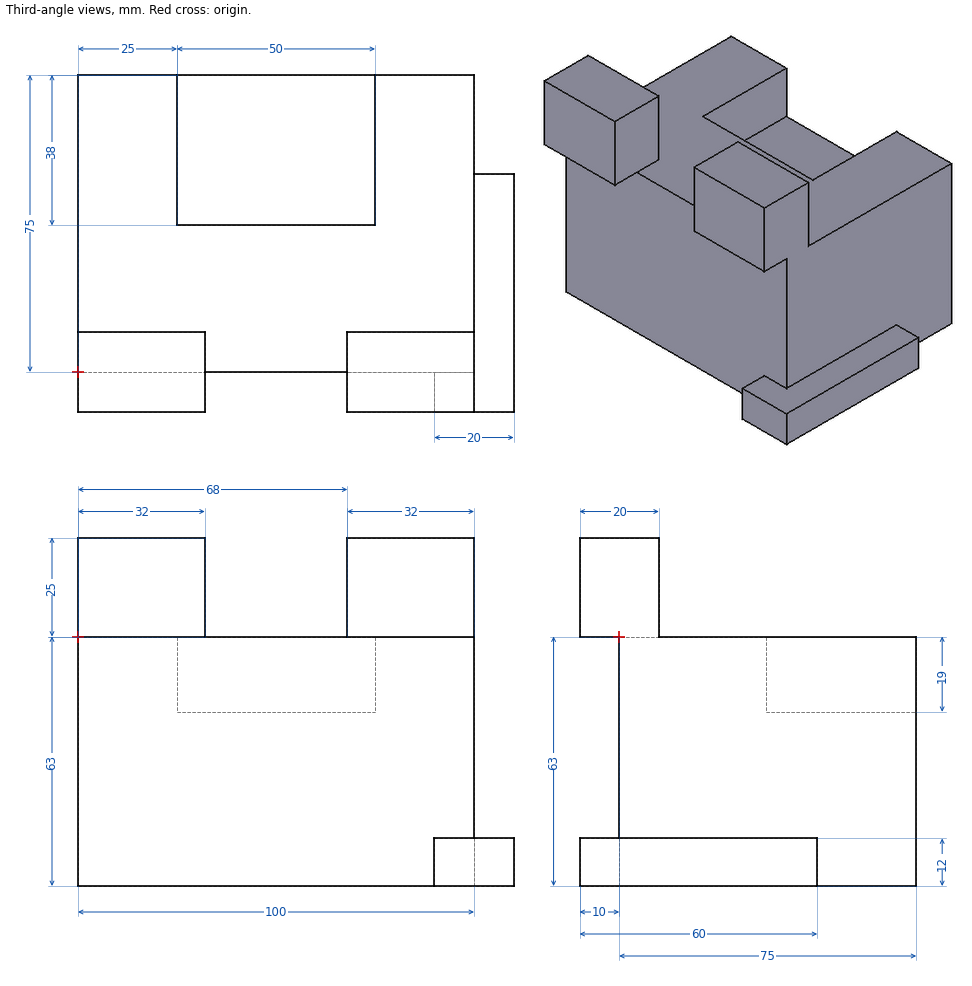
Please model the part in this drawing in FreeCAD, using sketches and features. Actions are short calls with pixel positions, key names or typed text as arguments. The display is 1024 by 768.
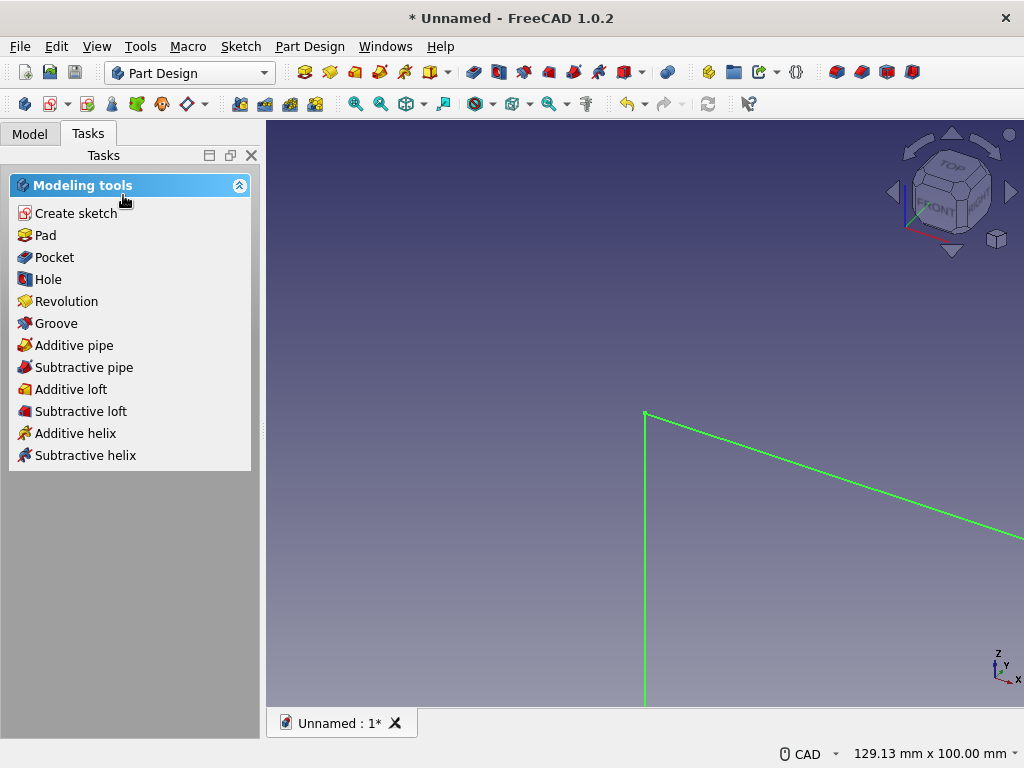
click(305, 72)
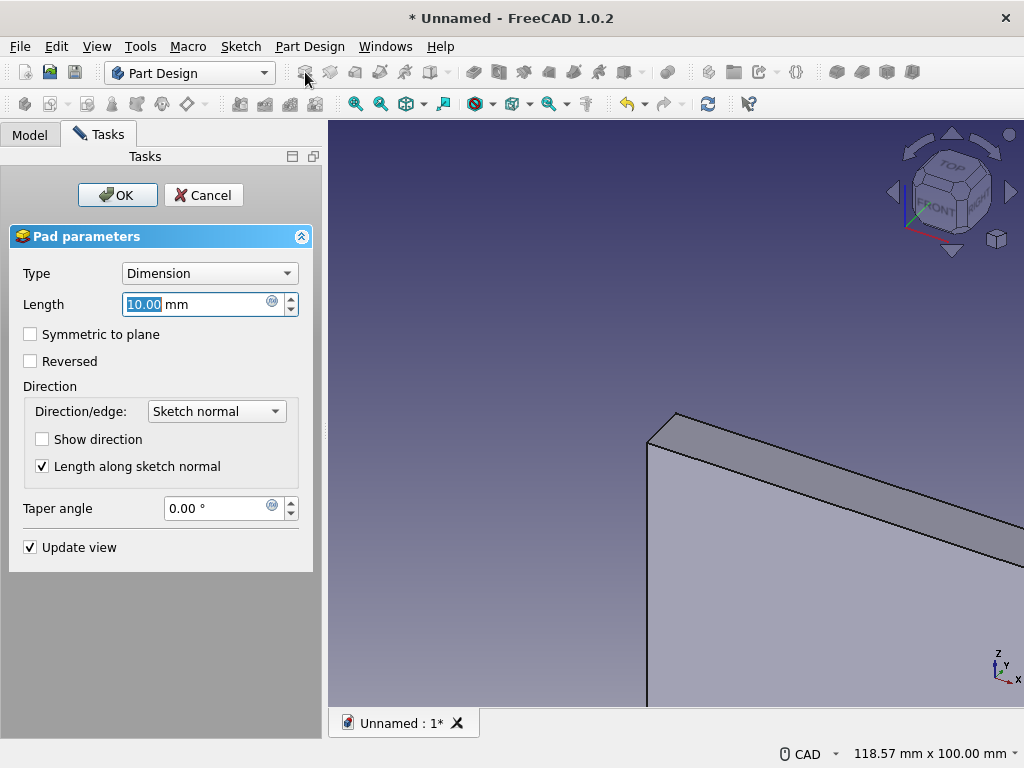
text(75)
key(Tab)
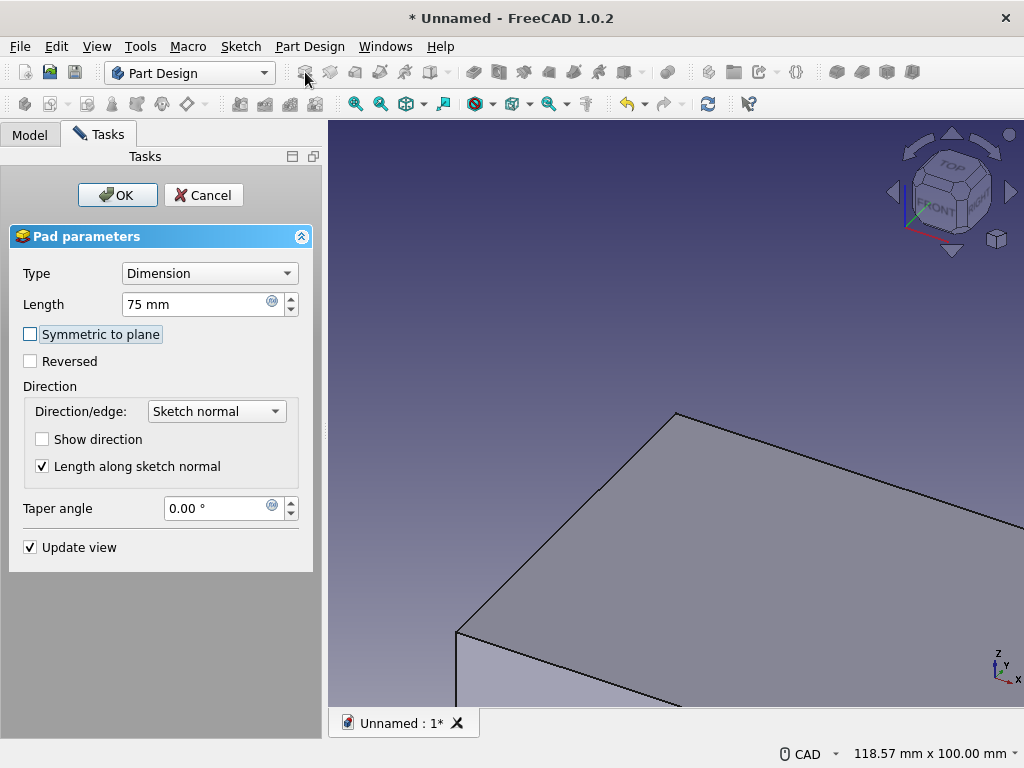
click(31, 361)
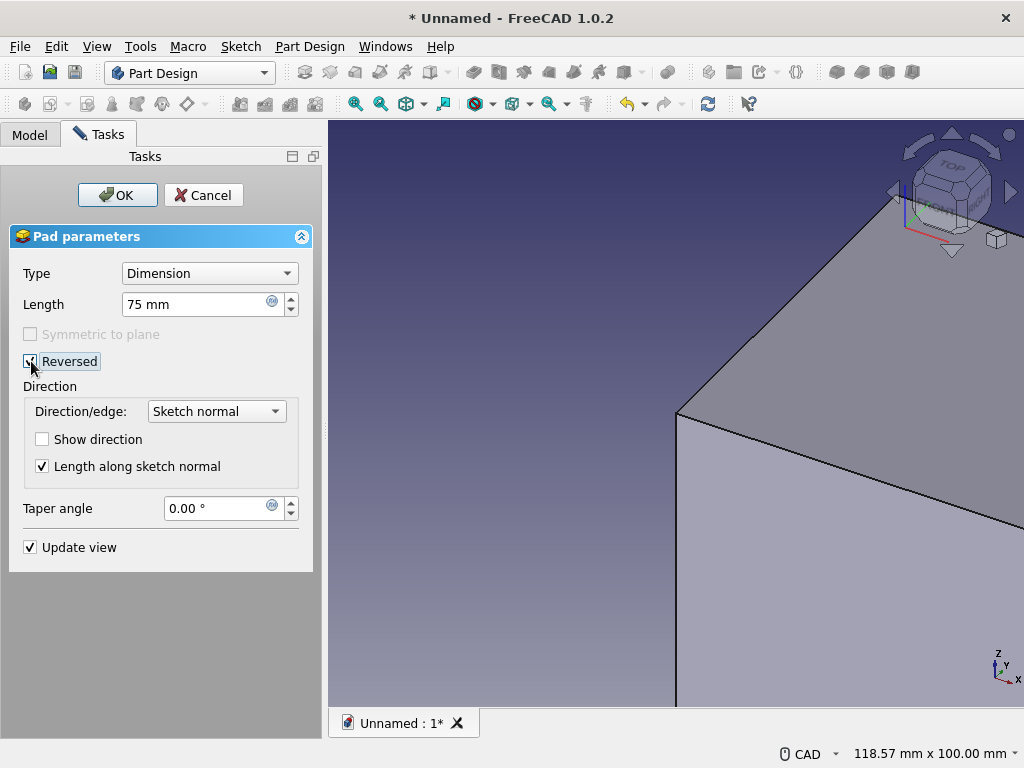
click(118, 195)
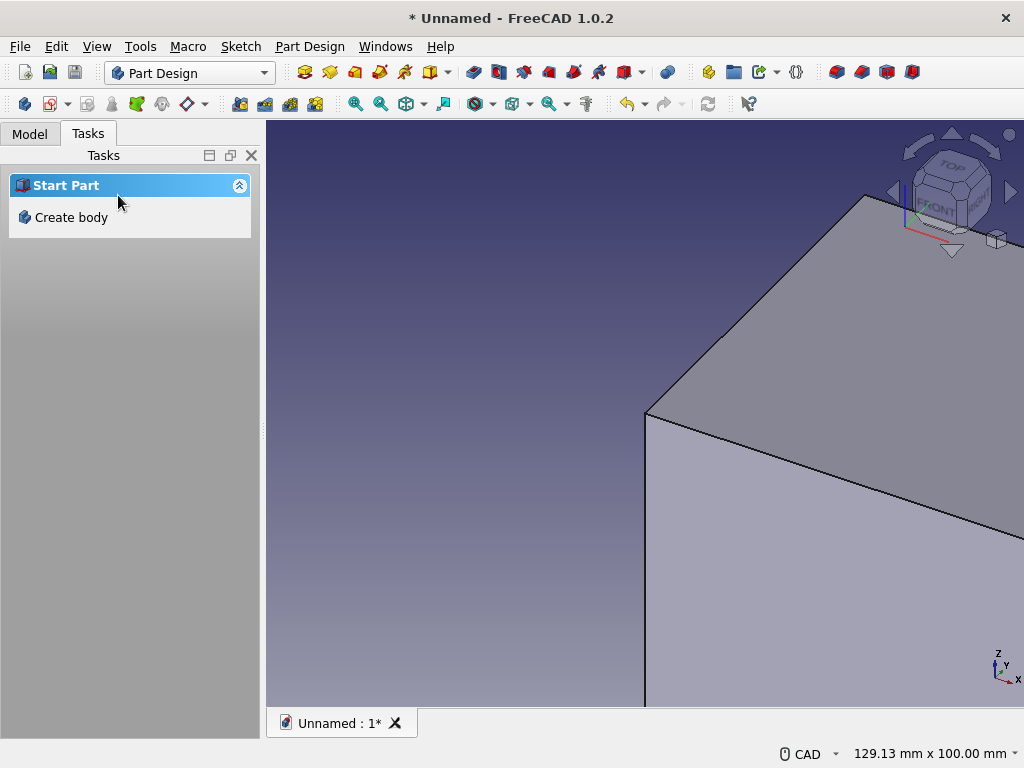
click(356, 104)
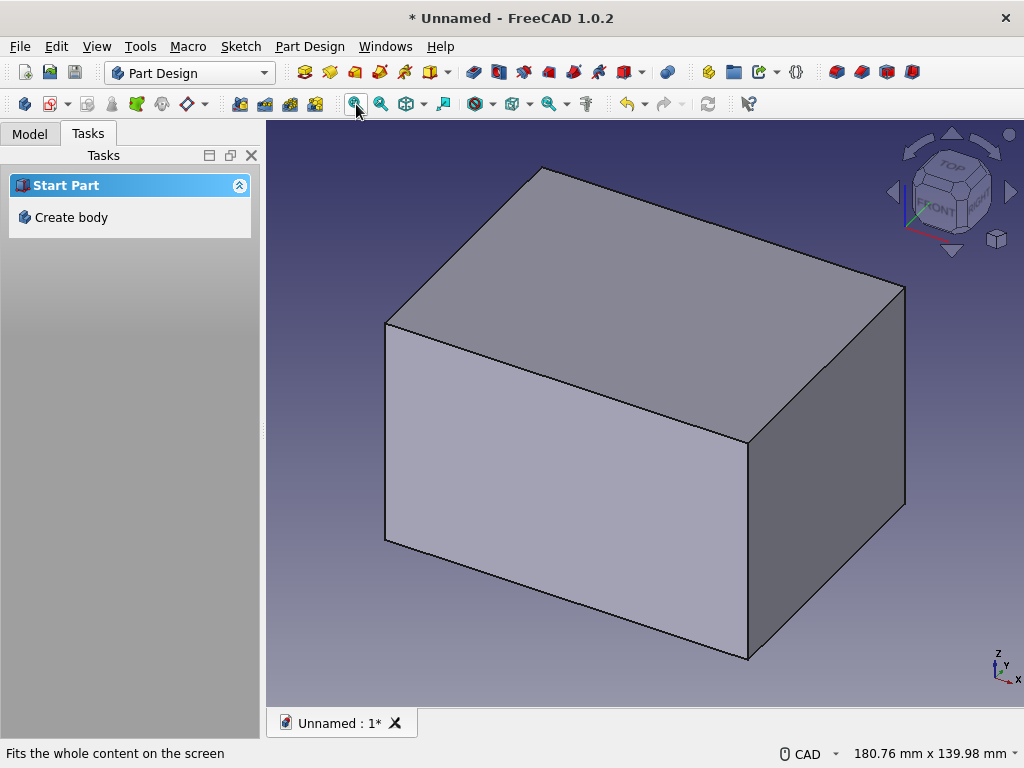
click(50, 104)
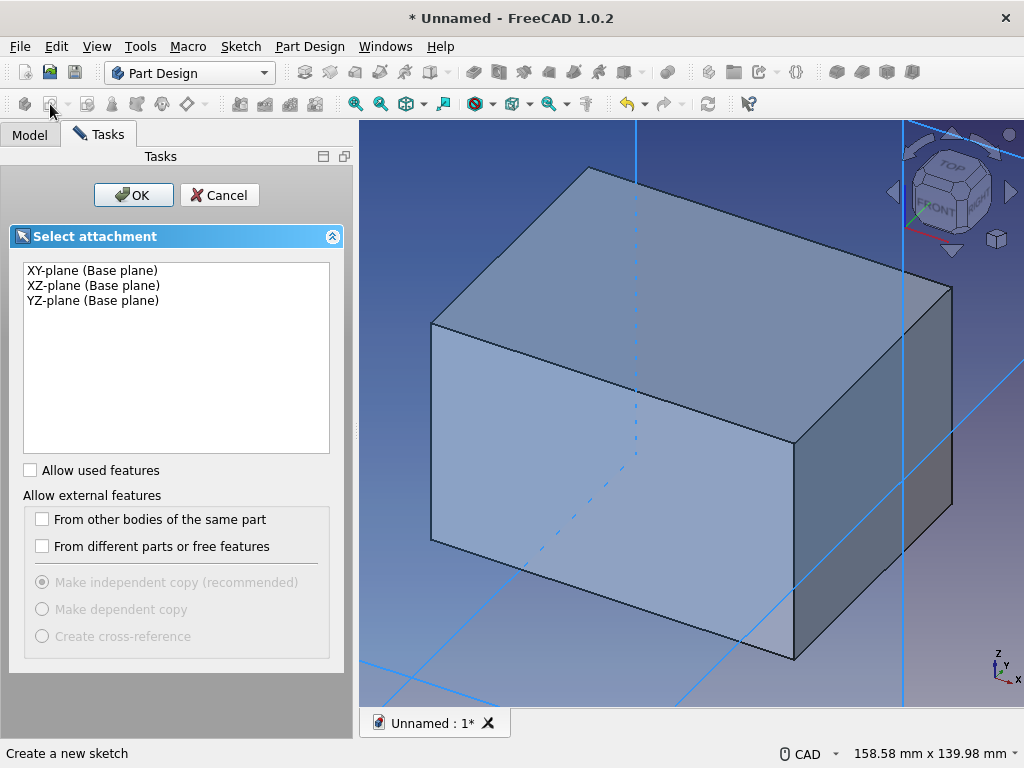
click(84, 270)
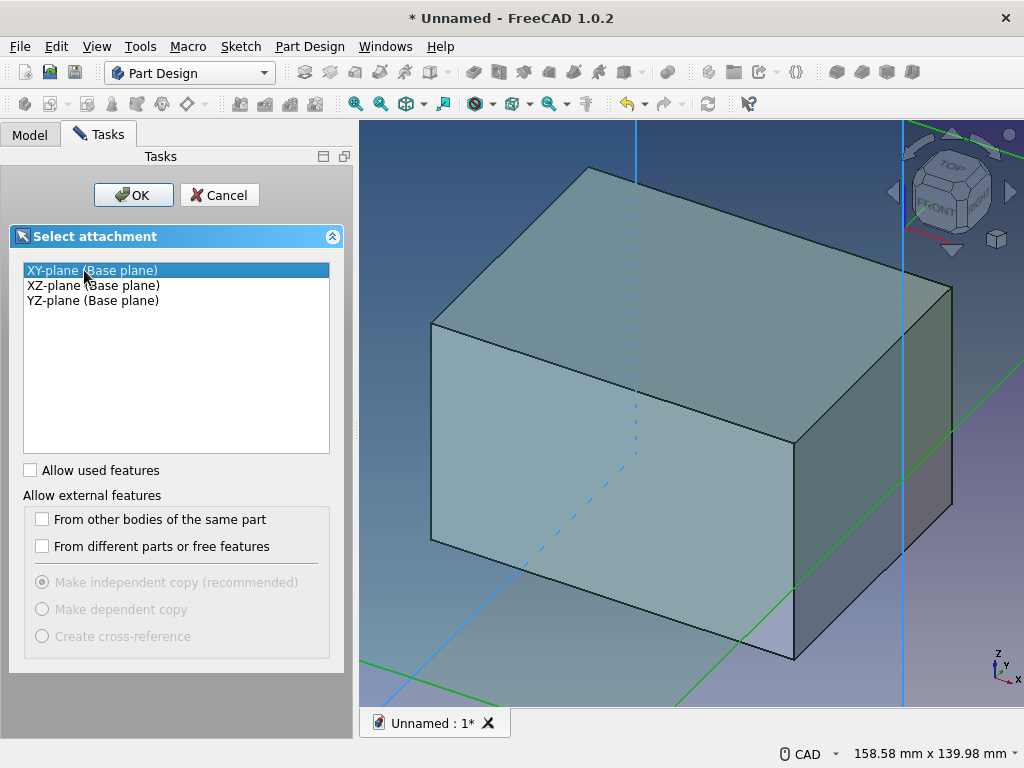
click(134, 195)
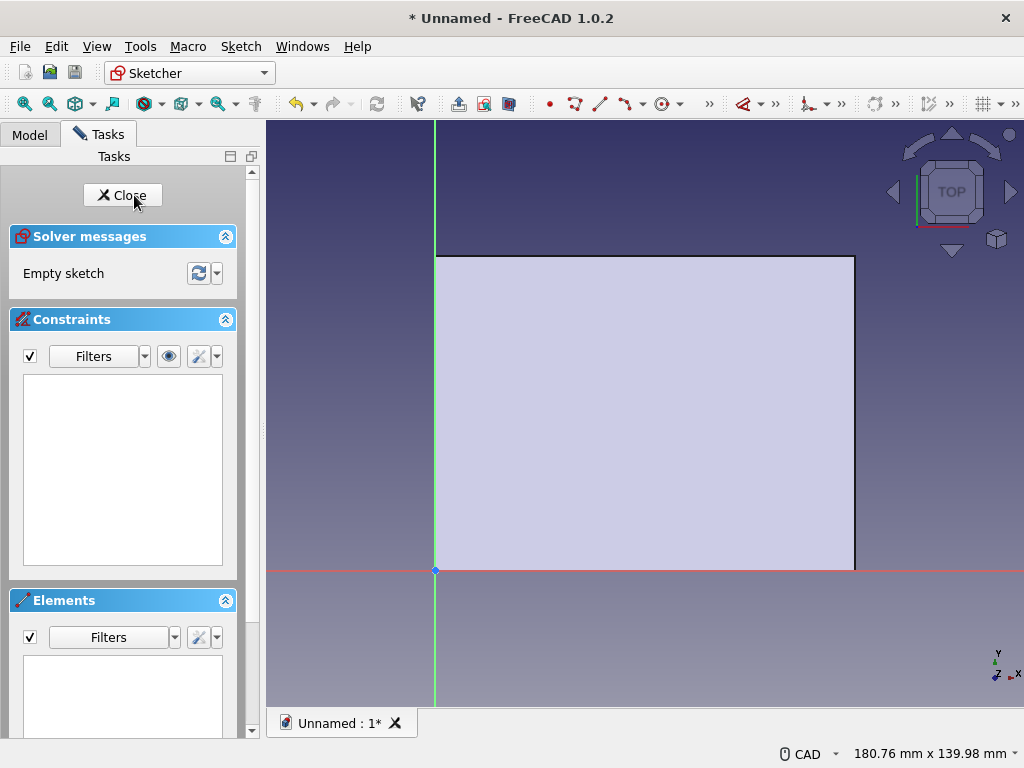
key(g)
key(r)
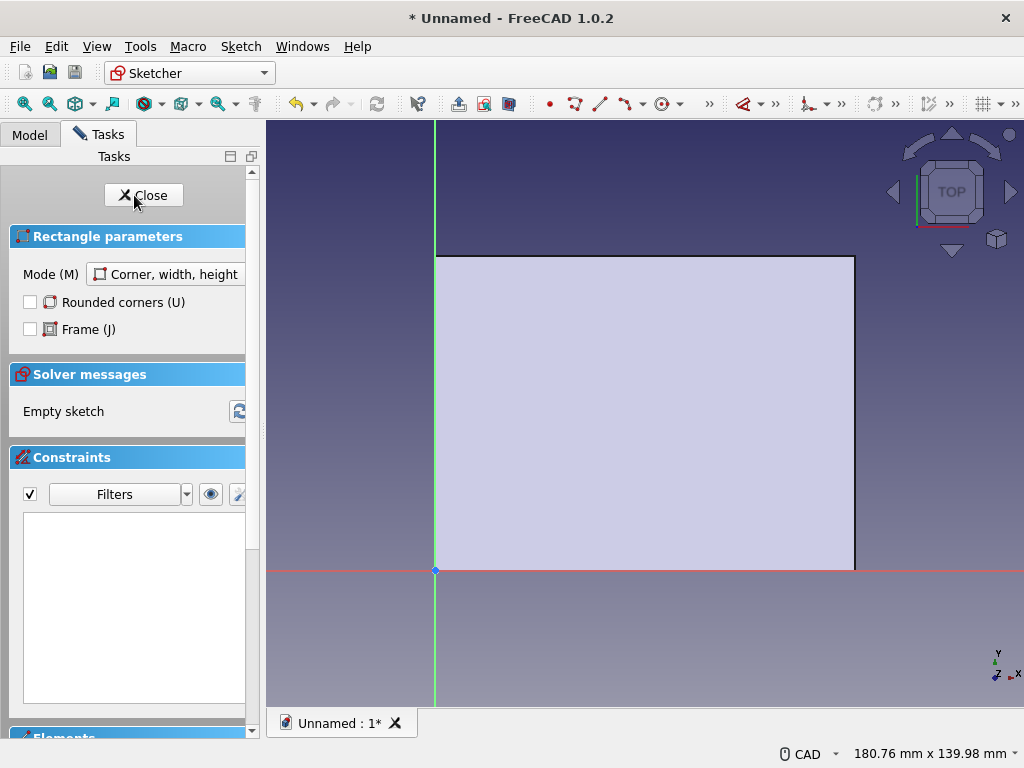
click(540, 256)
click(750, 416)
key(Escape)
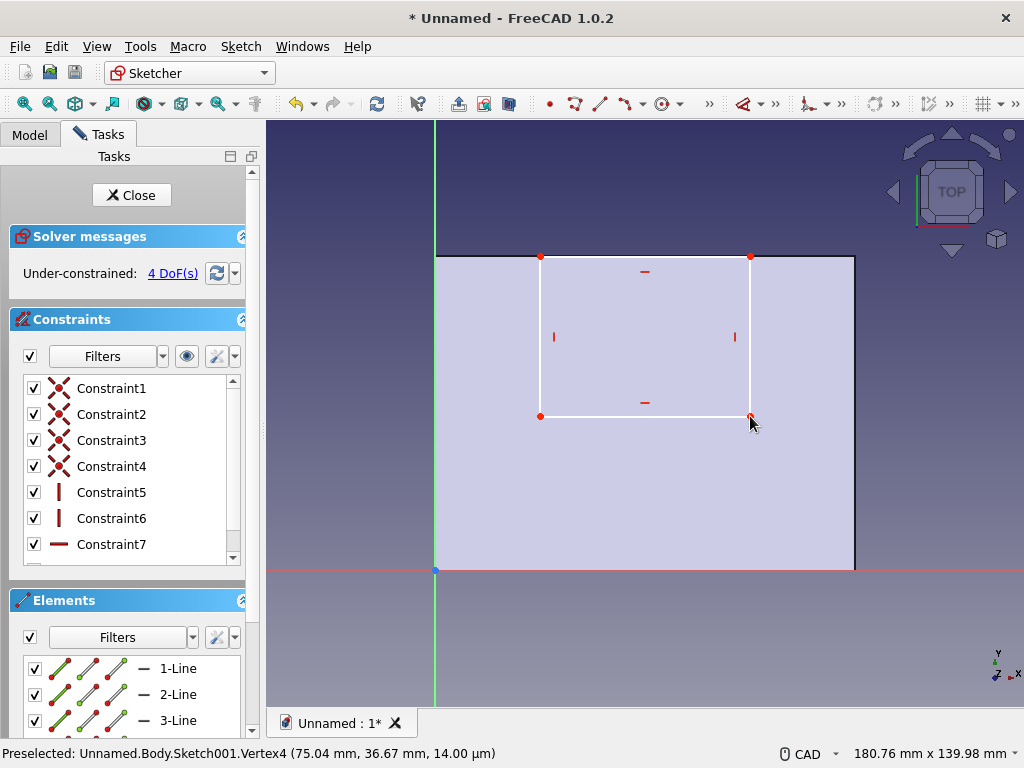
key(d)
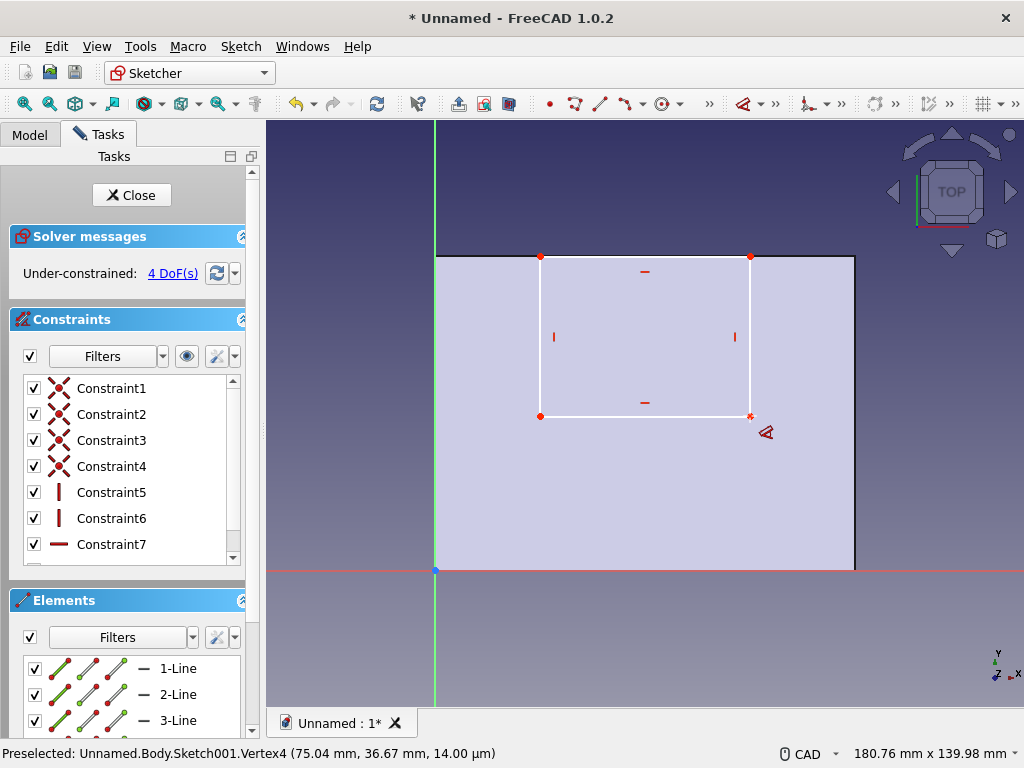
click(540, 305)
click(506, 337)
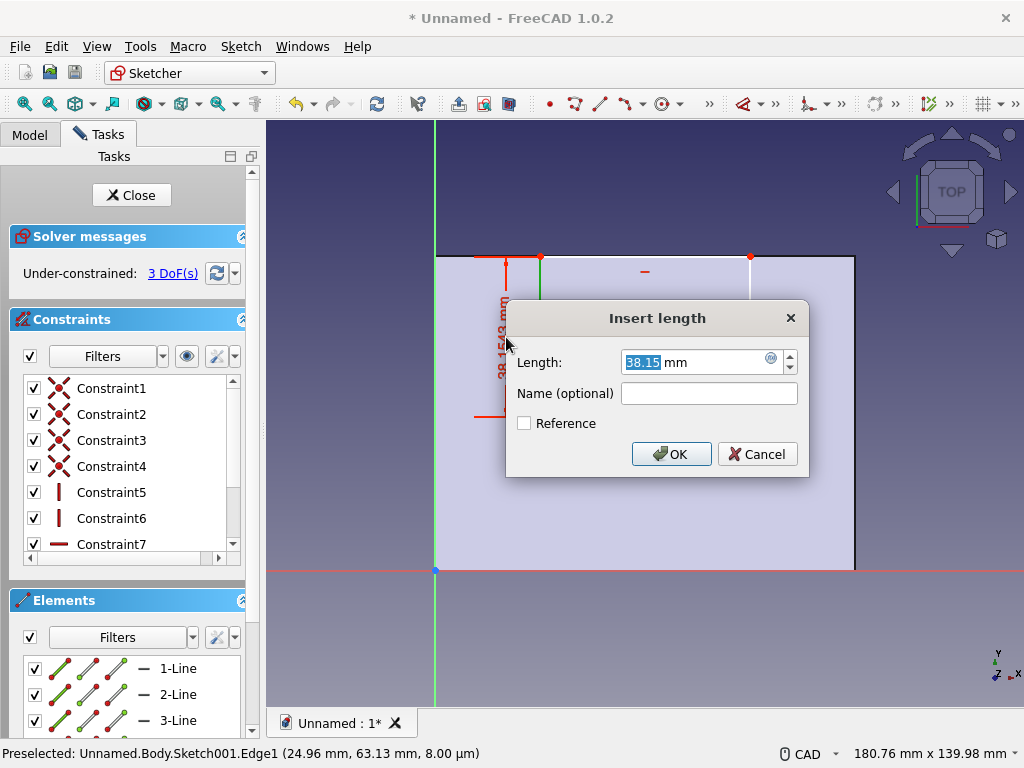
text(38)
key(Return)